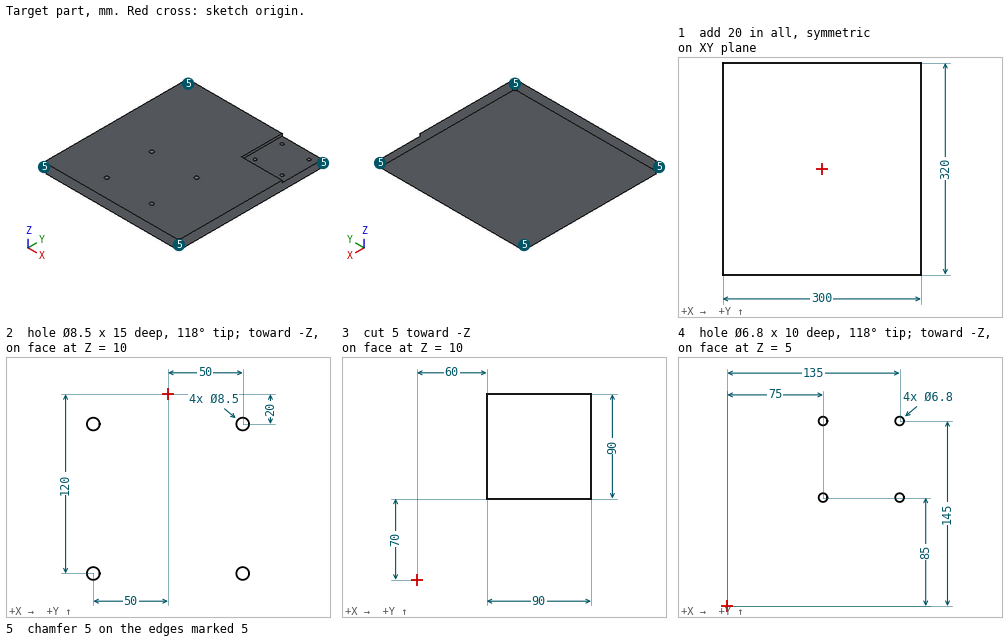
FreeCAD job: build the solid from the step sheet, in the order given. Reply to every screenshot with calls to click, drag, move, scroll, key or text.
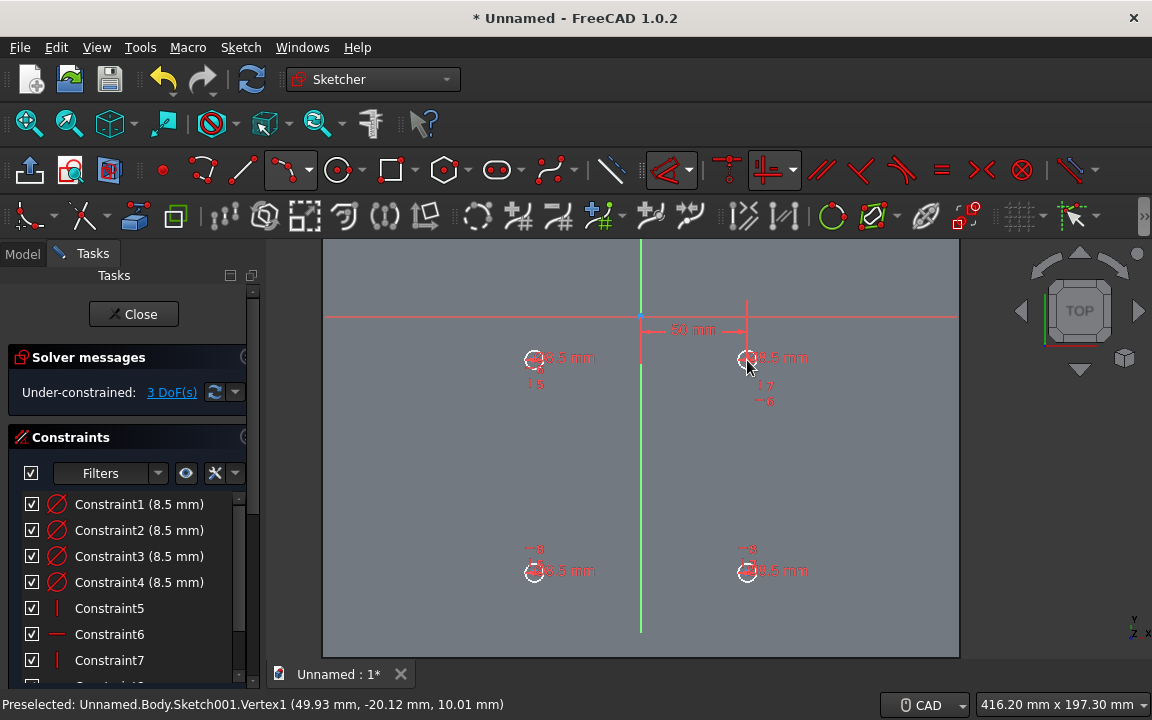
click(747, 360)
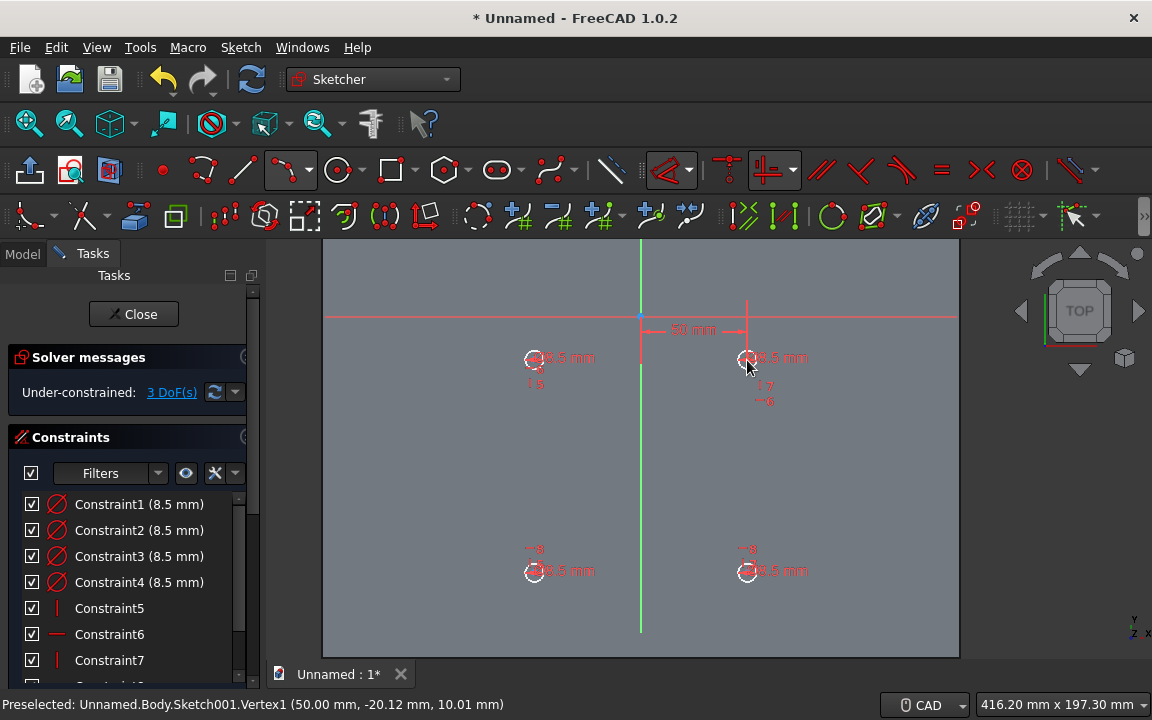
key(i)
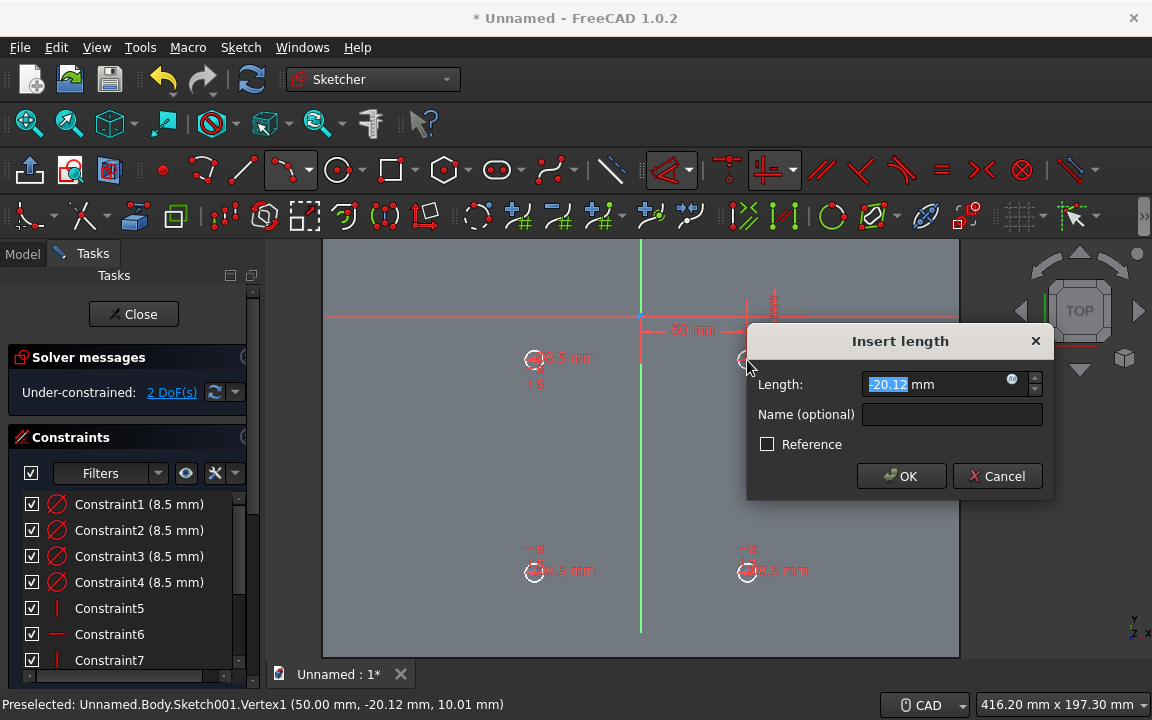
text(-20)
key(Return)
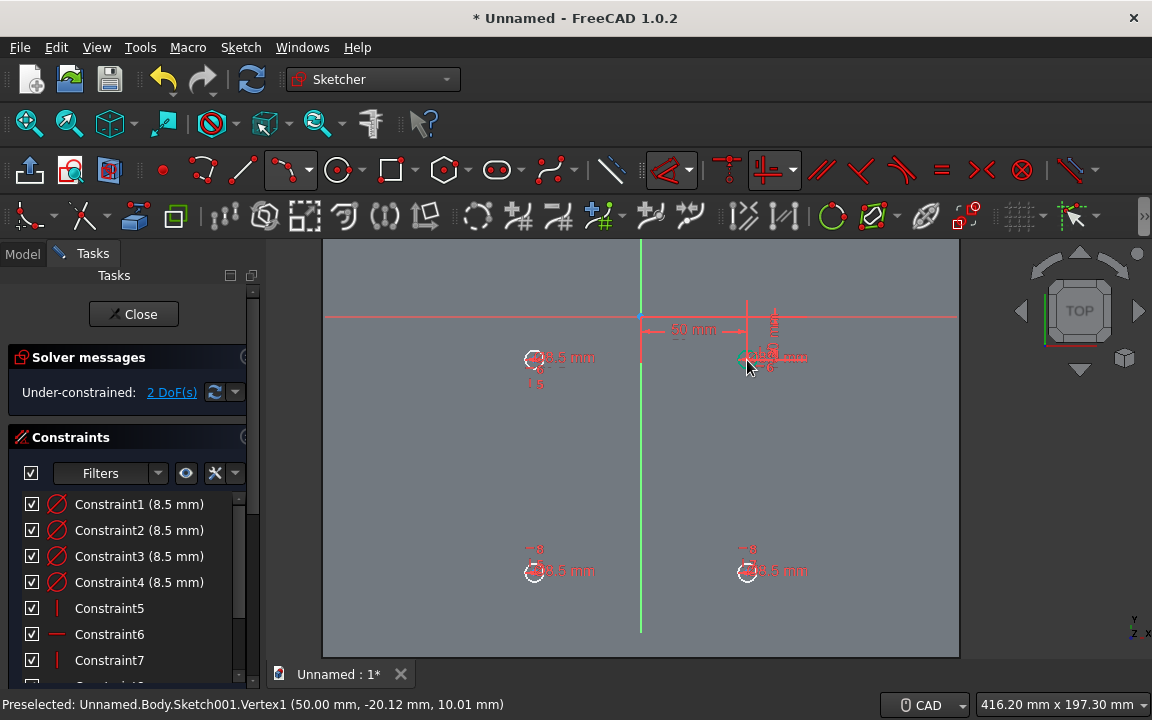
click(534, 573)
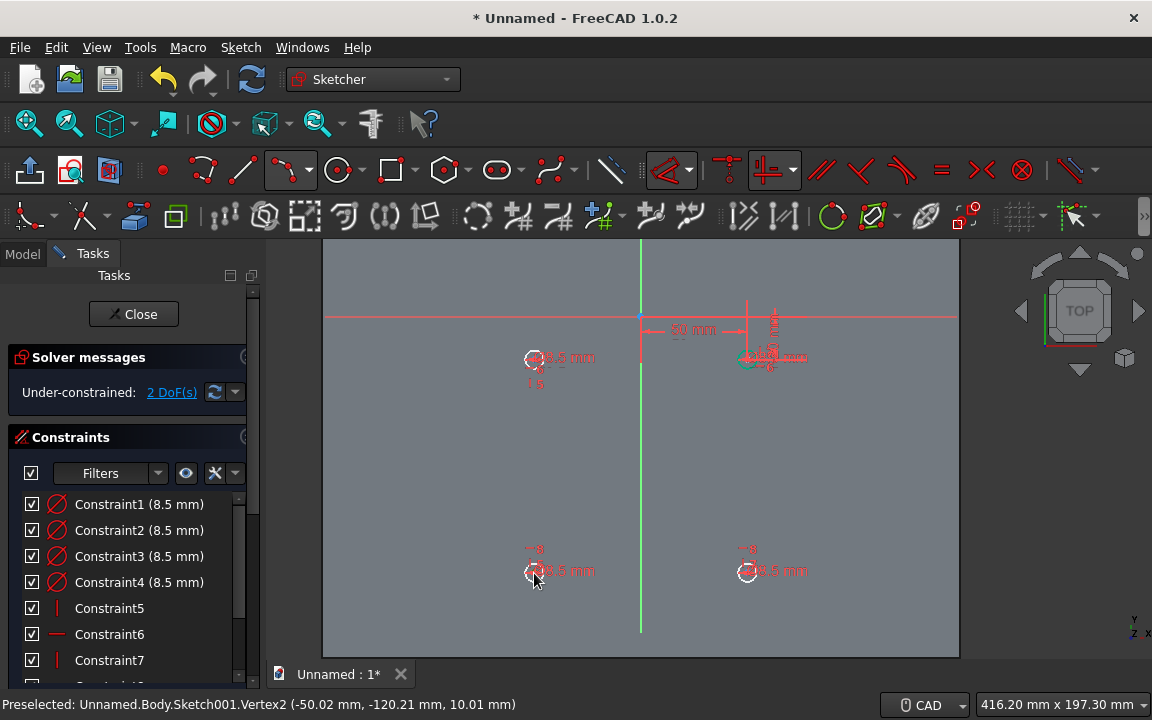
key(l)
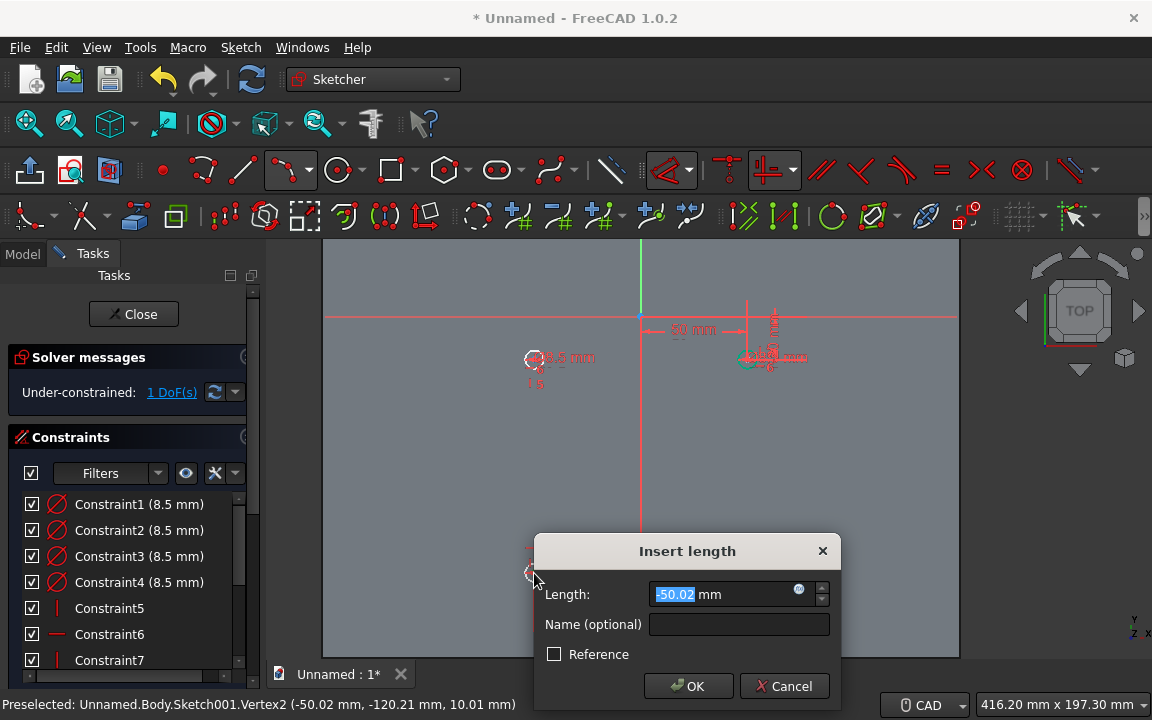
text(-50)
key(Return)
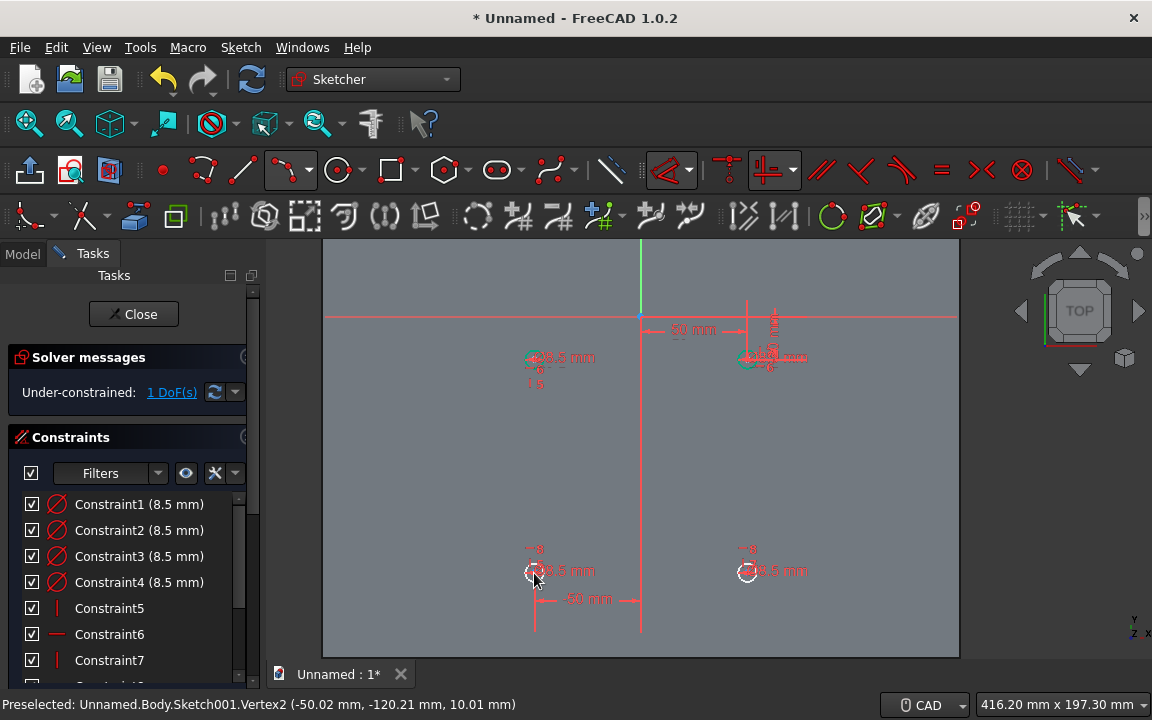
click(535, 573)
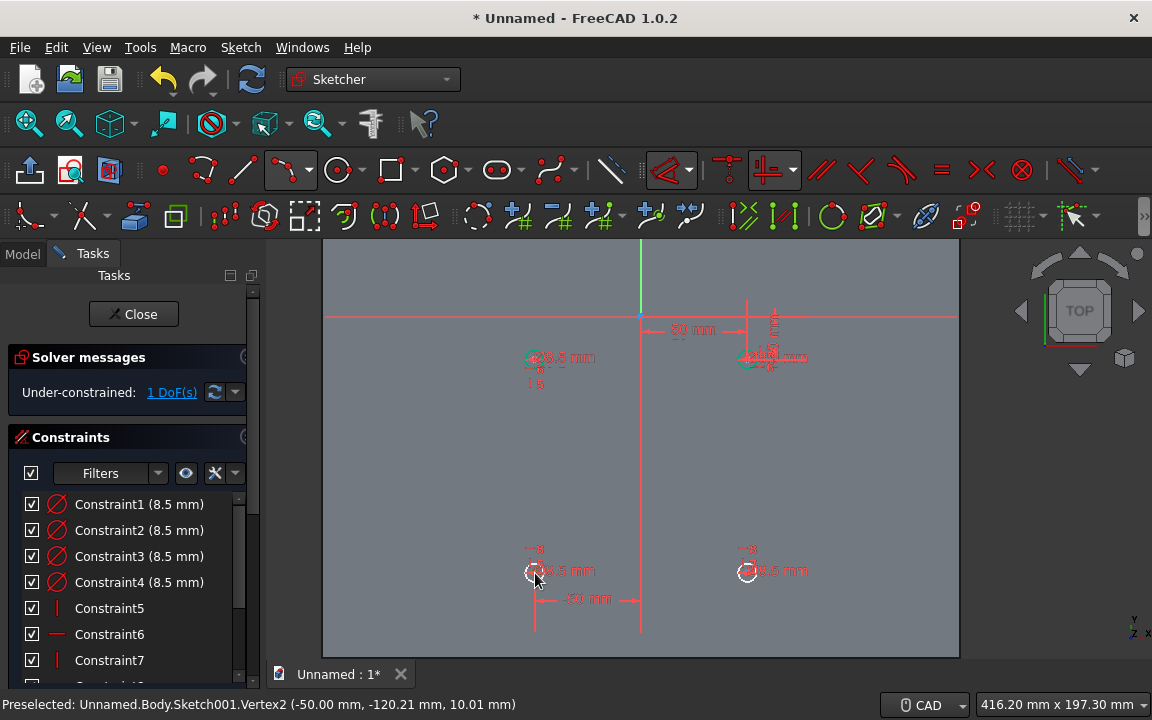
key(i)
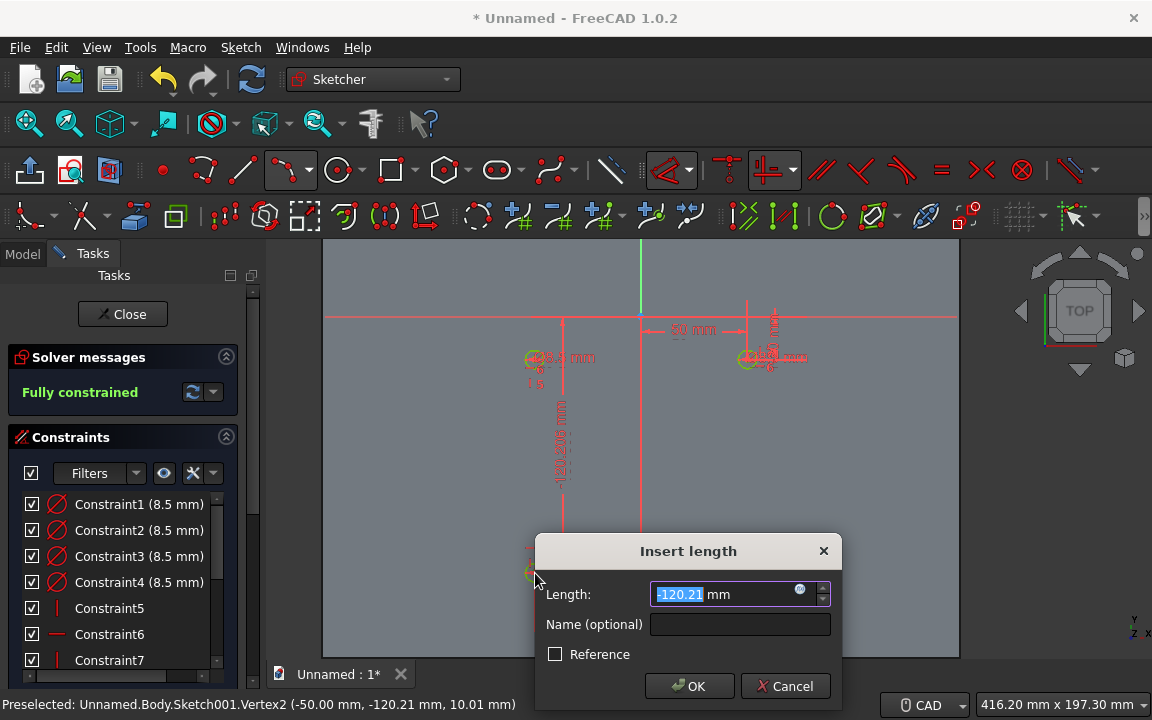
text(-120)
key(Return)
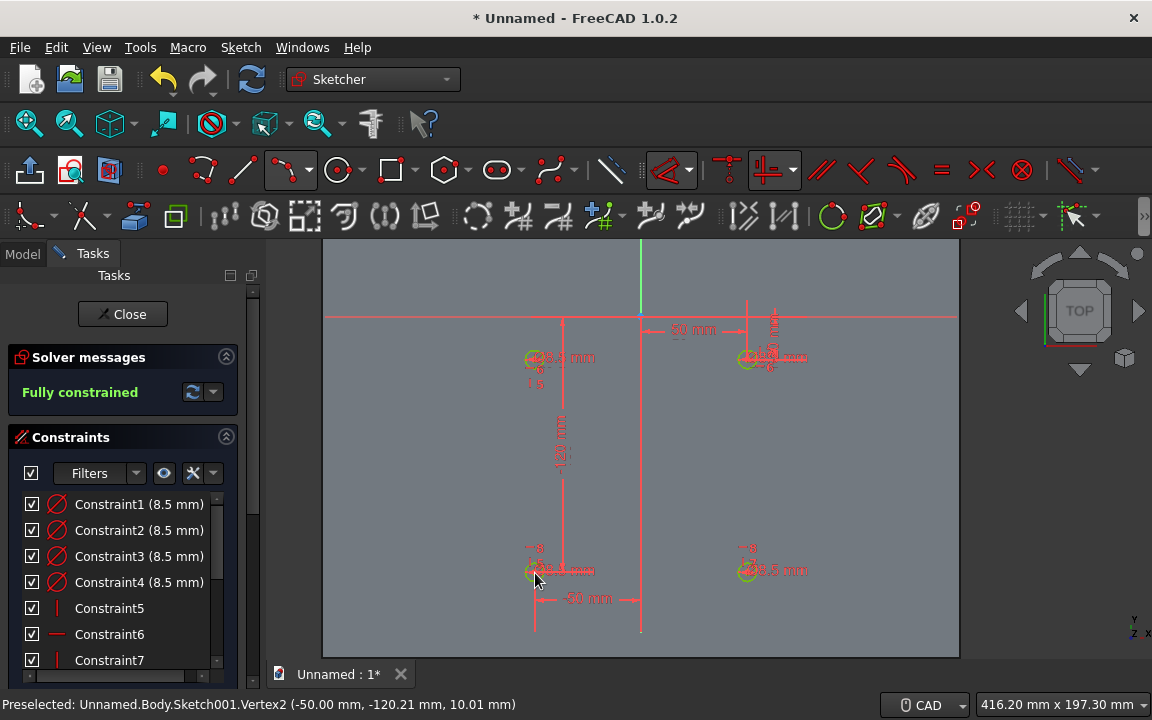
click(123, 314)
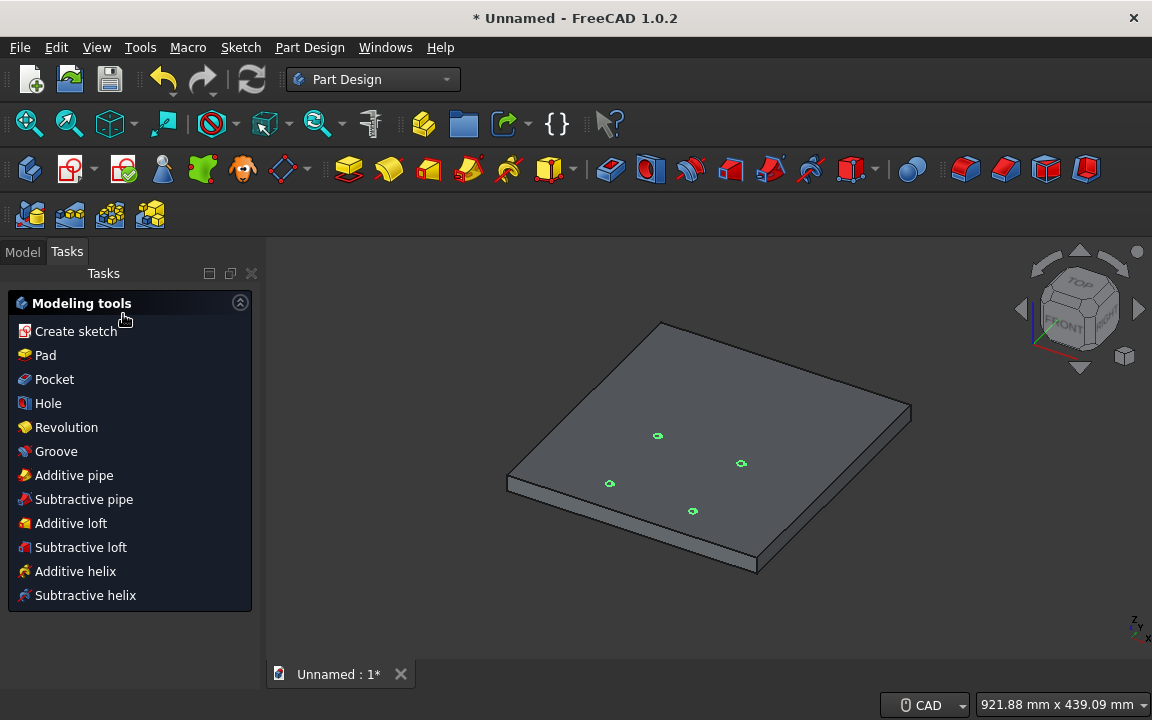
click(652, 170)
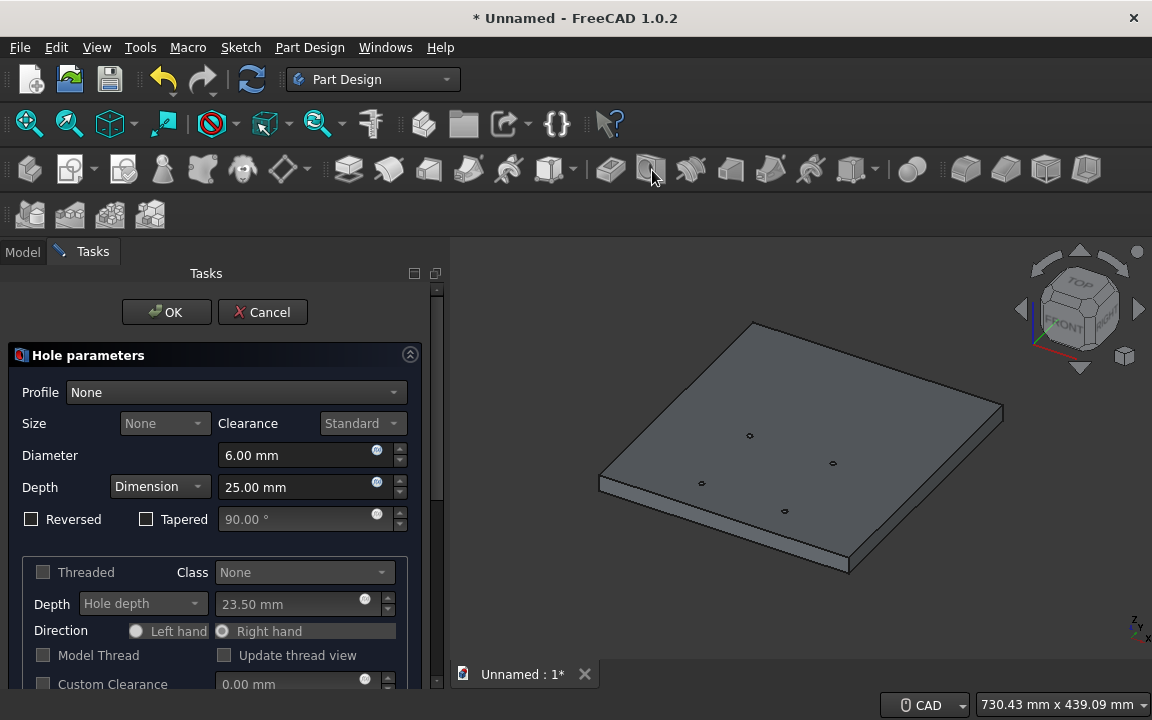
triple_click(305, 455)